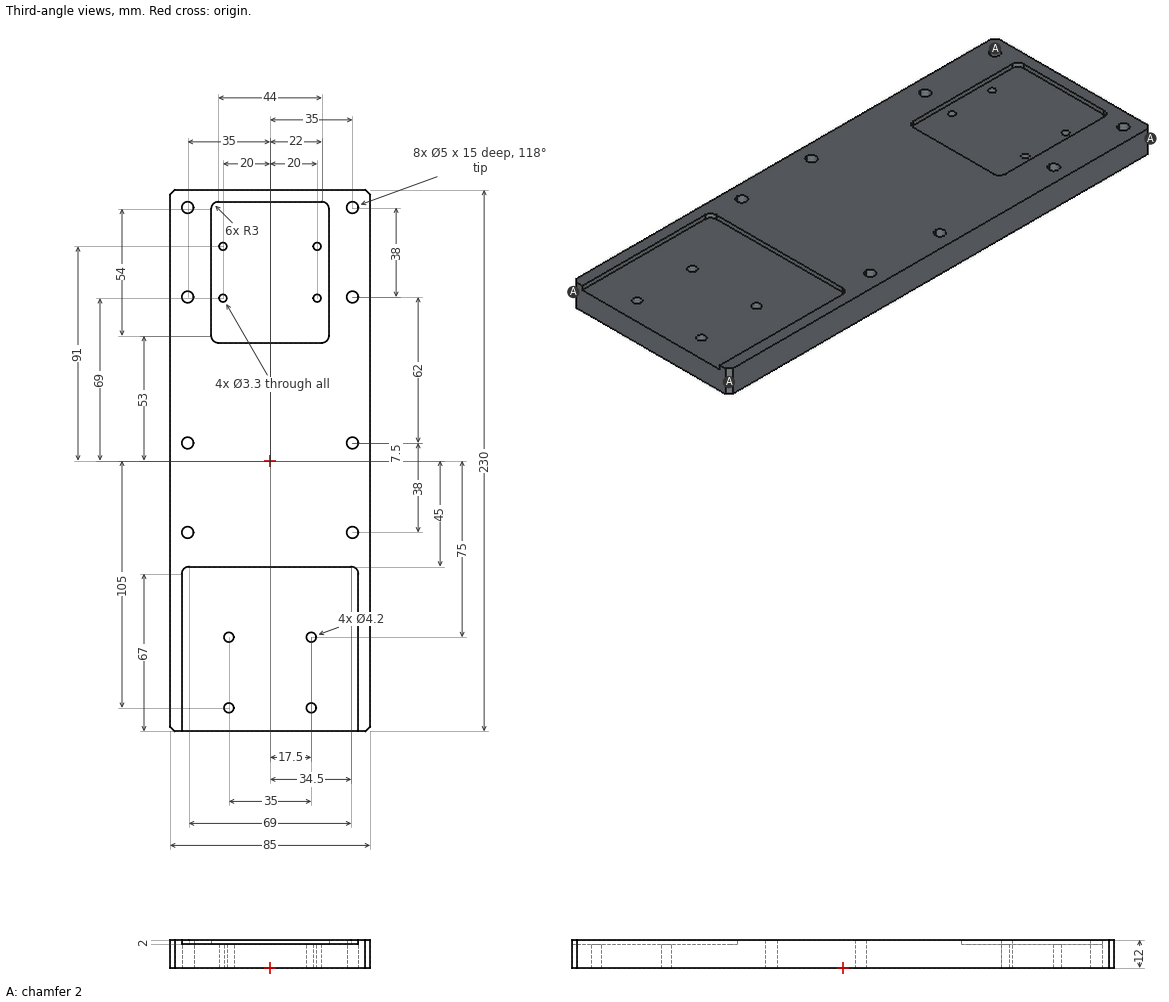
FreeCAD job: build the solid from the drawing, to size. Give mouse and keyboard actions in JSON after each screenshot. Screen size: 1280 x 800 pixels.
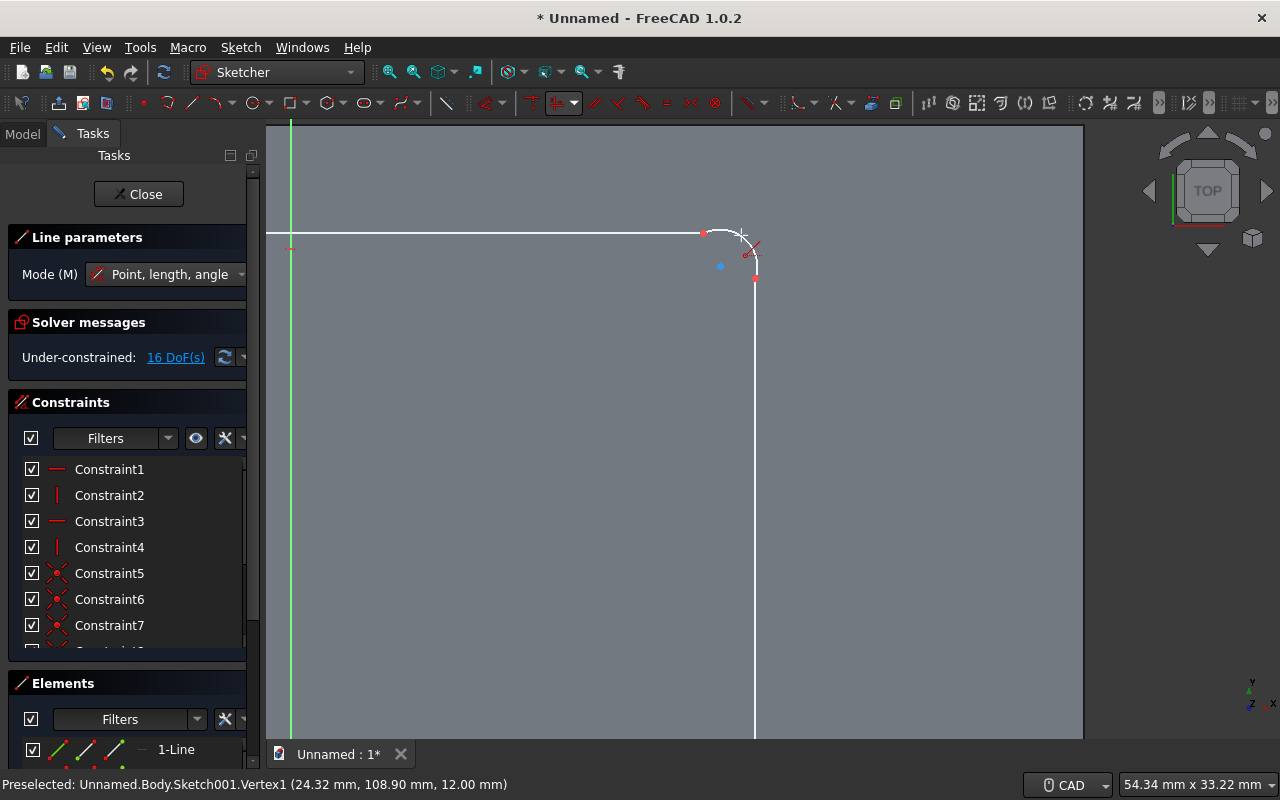
{"action": "scroll", "coordinate": [746, 241], "scroll_direction": "down", "scroll_amount": 12}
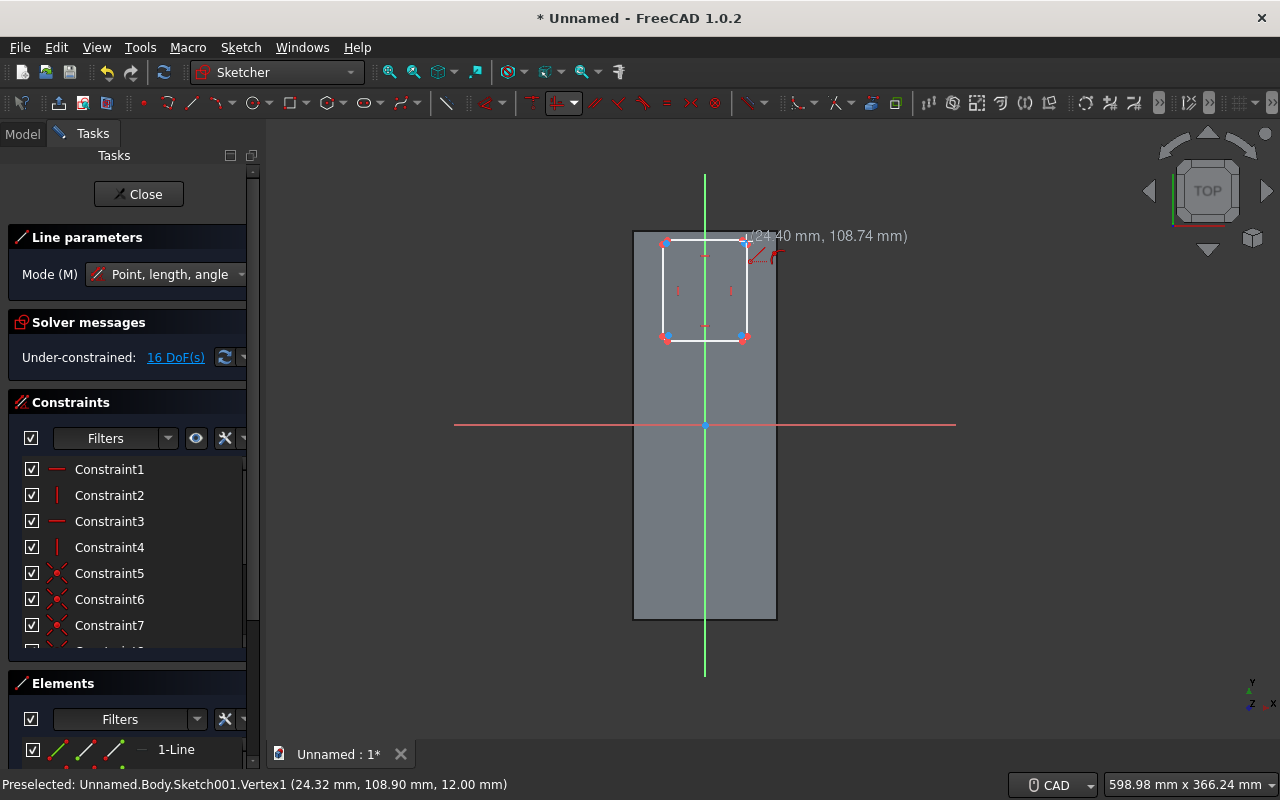
{"action": "left_click", "coordinate": [764, 502]}
{"action": "left_click", "coordinate": [647, 502]}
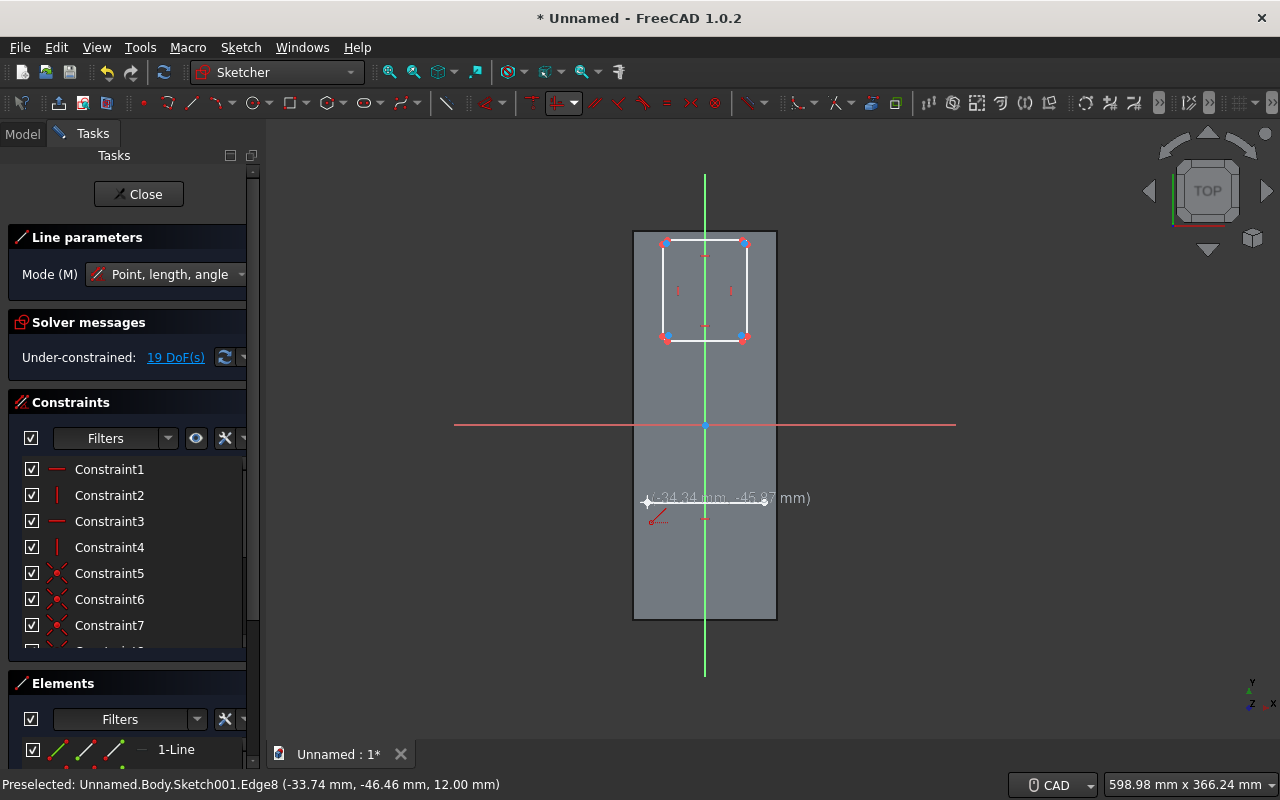
{"action": "key", "text": "g m"}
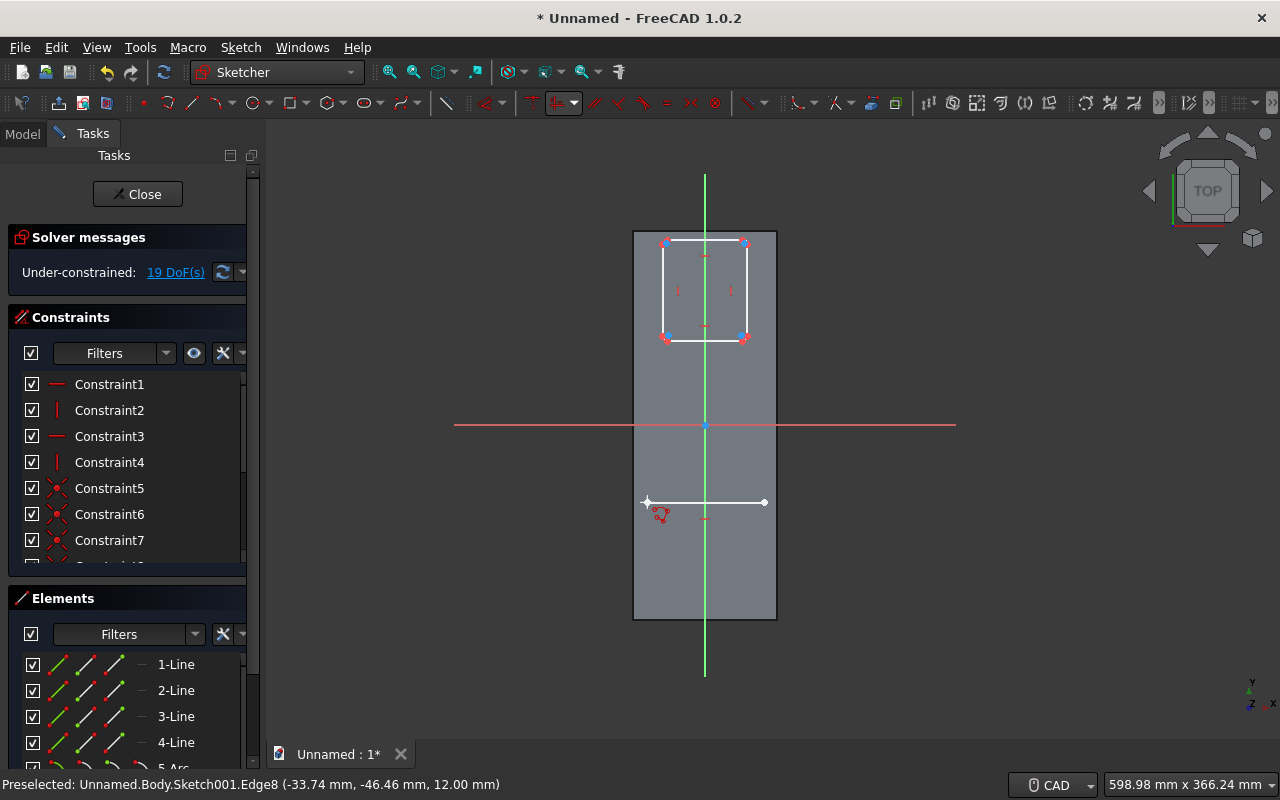
{"action": "scroll", "coordinate": [642, 507], "scroll_direction": "up", "scroll_amount": 4}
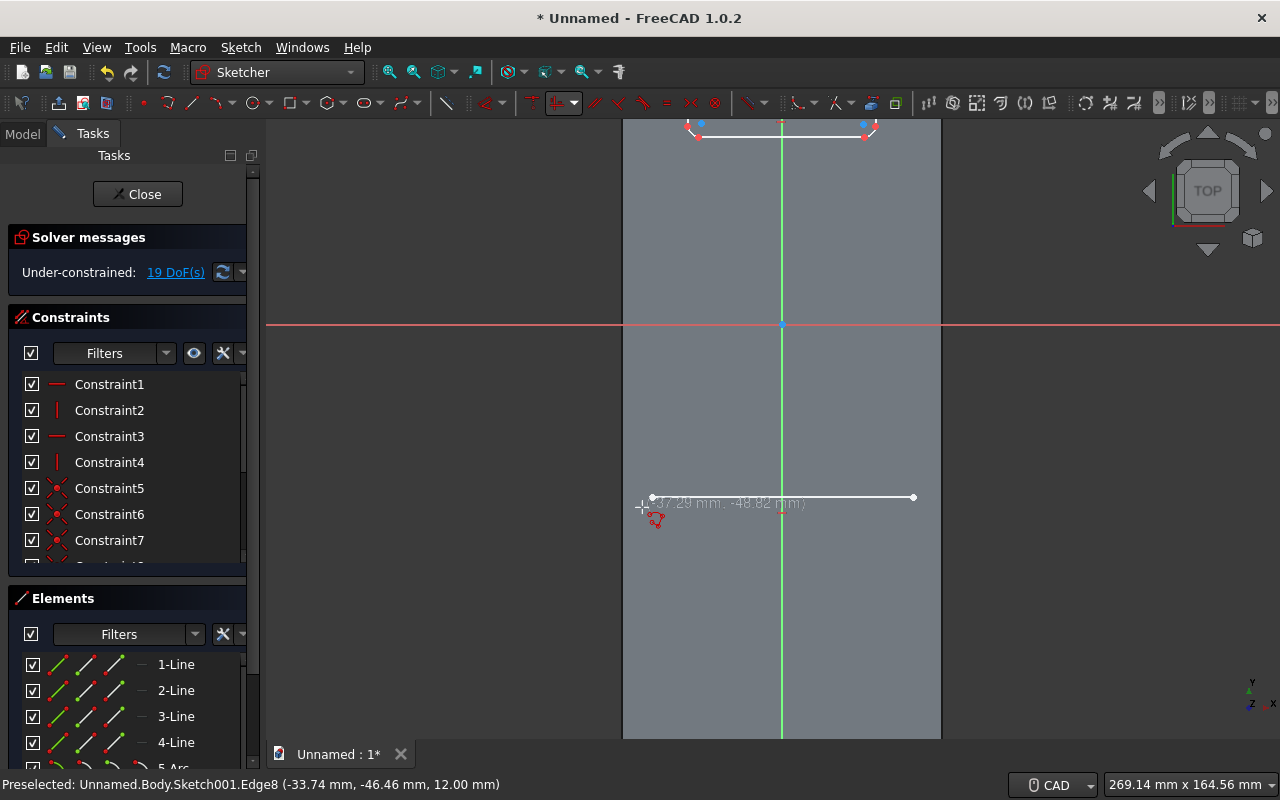
{"action": "left_click", "coordinate": [641, 505]}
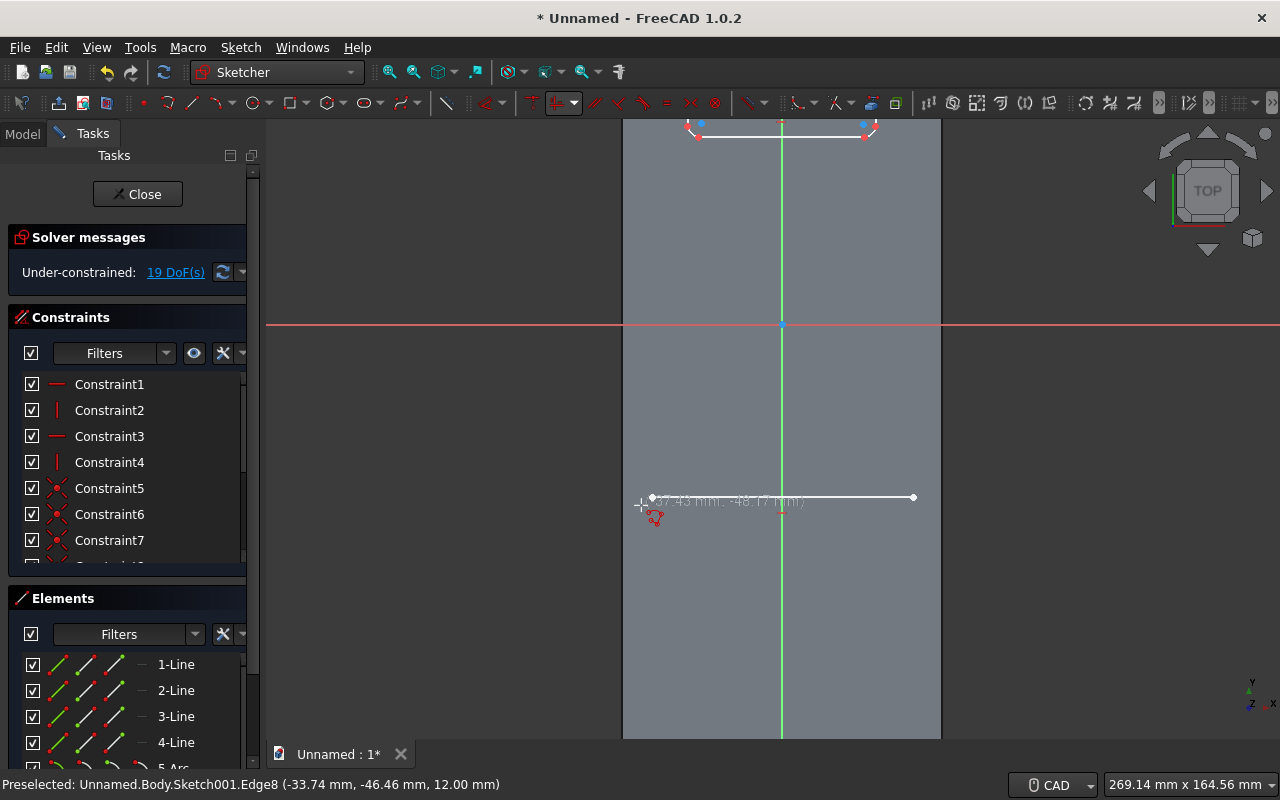
{"action": "scroll", "coordinate": [641, 507], "scroll_direction": "down", "scroll_amount": 4}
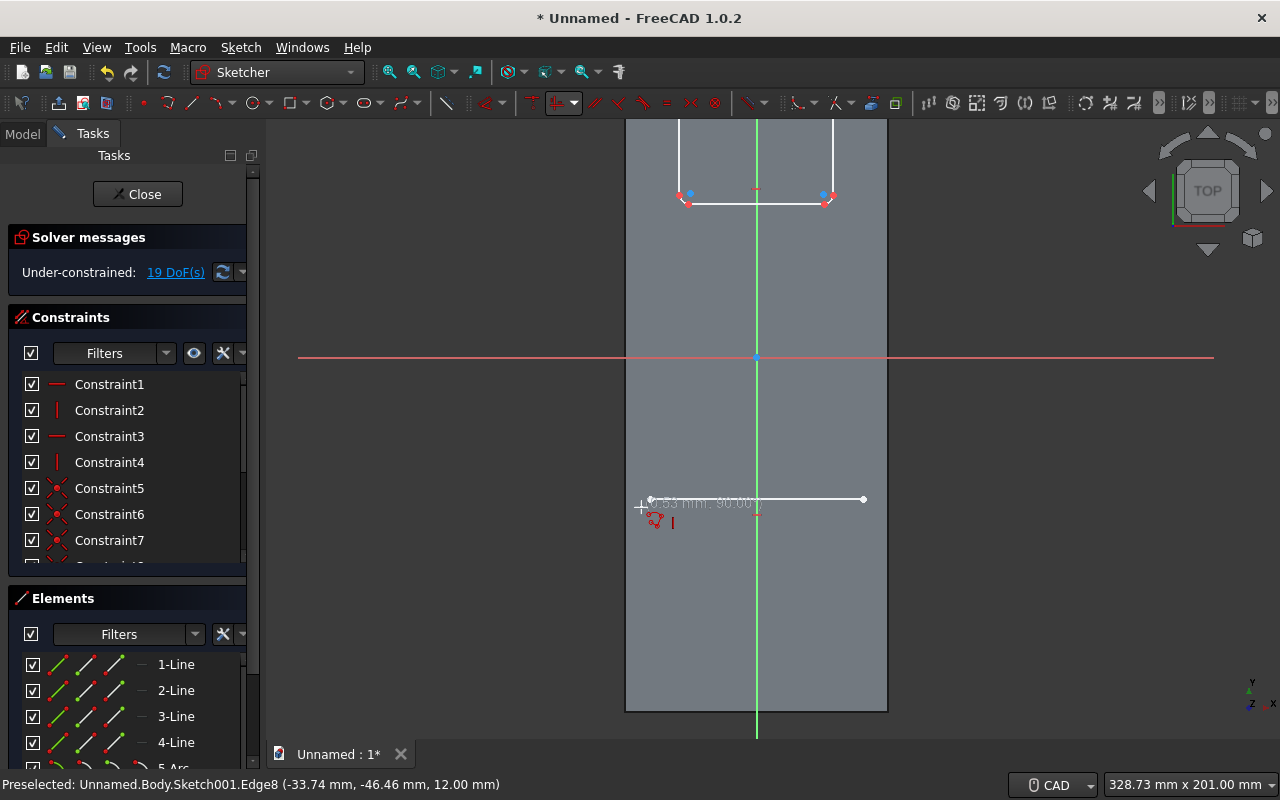
{"action": "left_click", "coordinate": [641, 620]}
{"action": "left_click", "coordinate": [768, 620]}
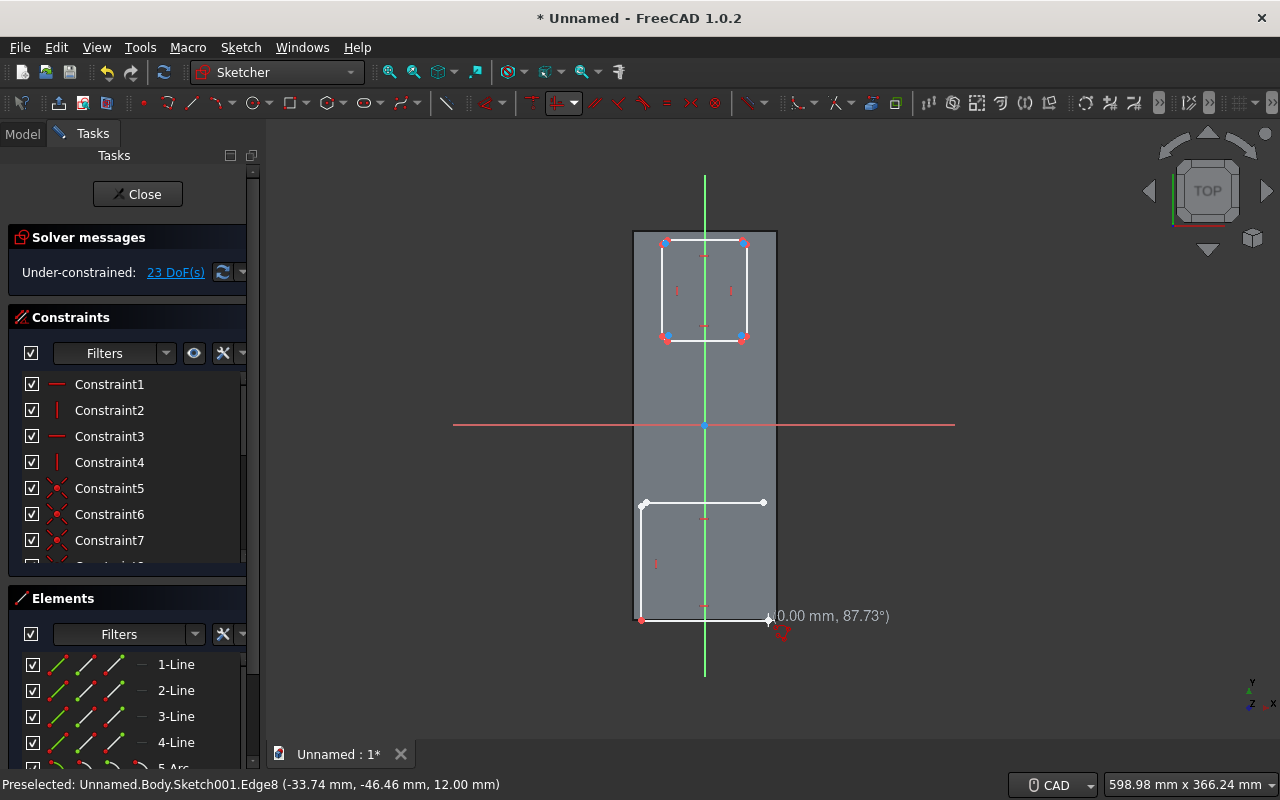
{"action": "scroll", "coordinate": [768, 507], "scroll_direction": "up", "scroll_amount": 4}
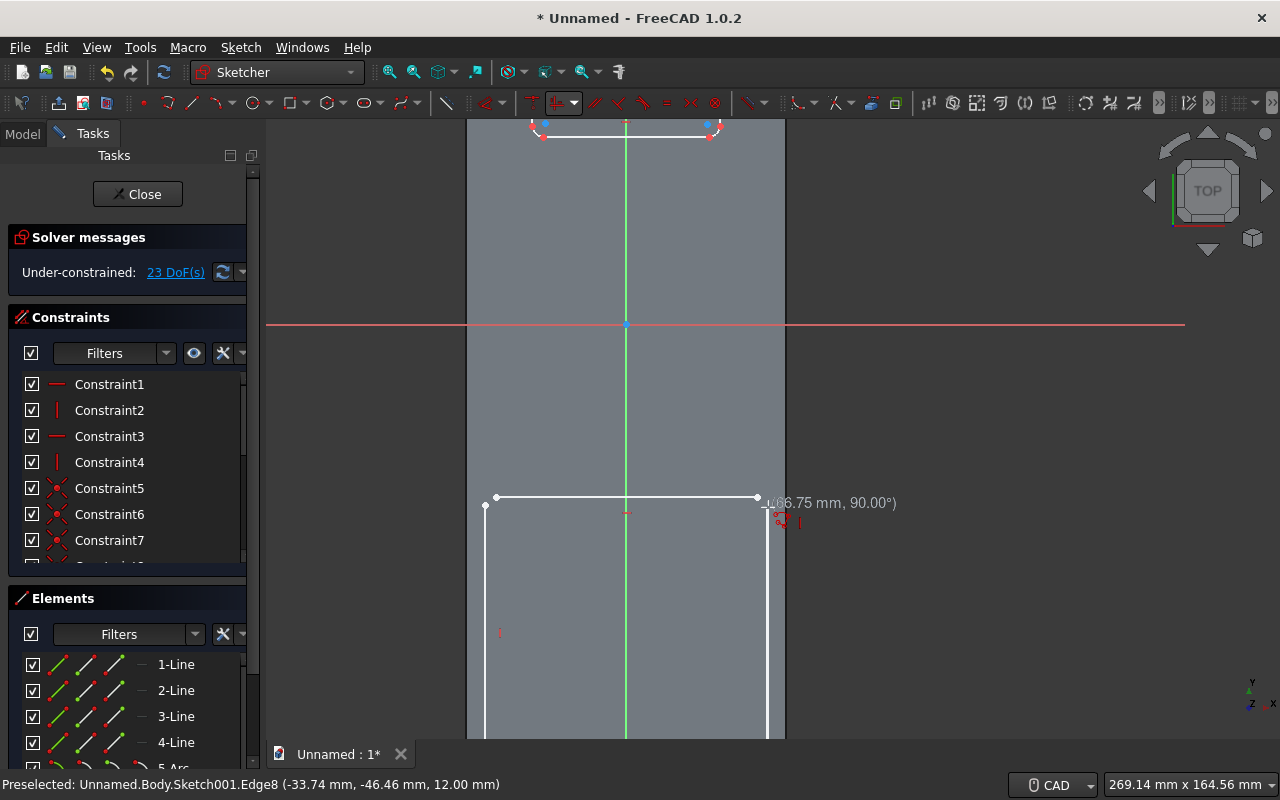
{"action": "left_click", "coordinate": [767, 505]}
{"action": "right_click", "coordinate": [767, 505]}